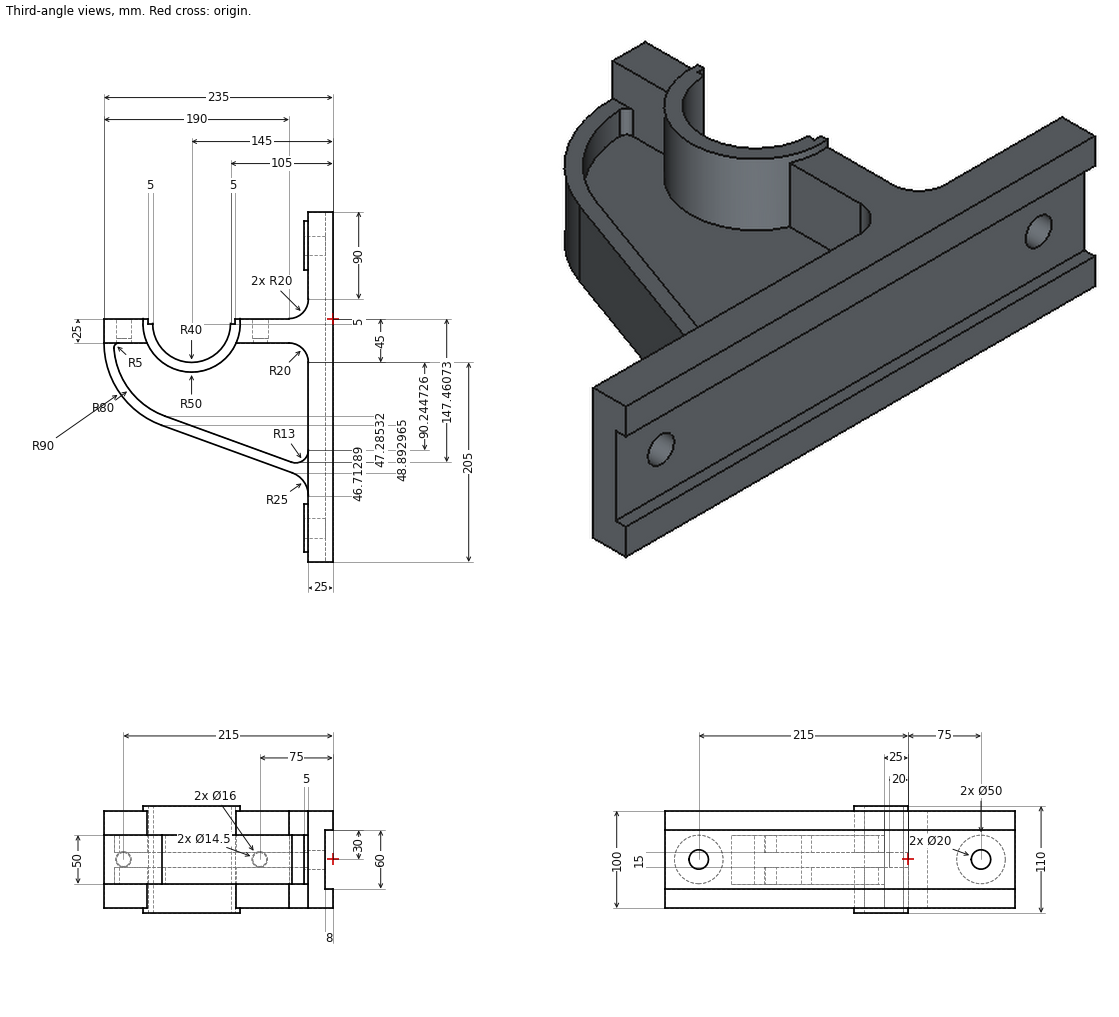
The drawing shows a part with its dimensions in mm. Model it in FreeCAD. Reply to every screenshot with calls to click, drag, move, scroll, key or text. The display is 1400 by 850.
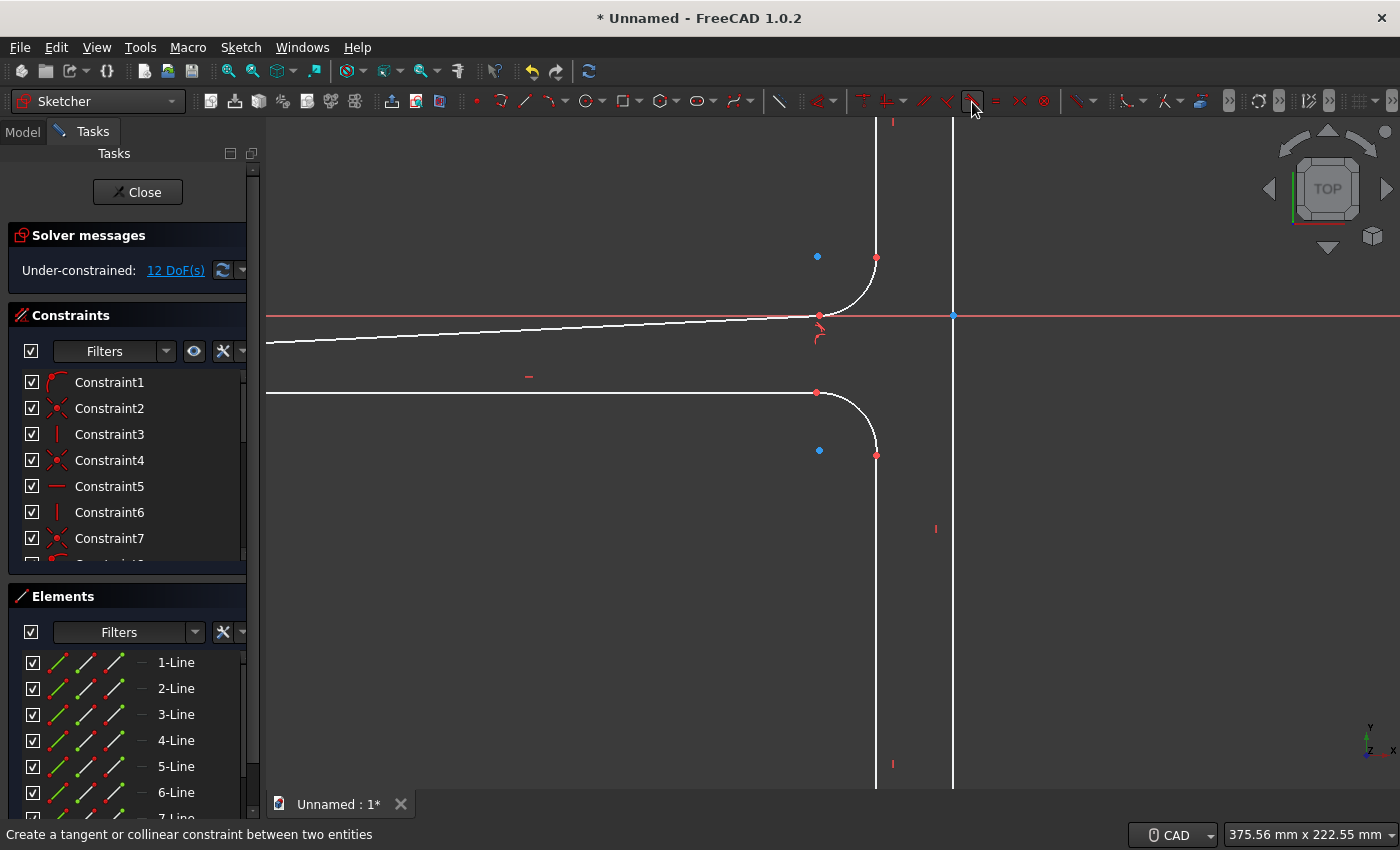
click(415, 393)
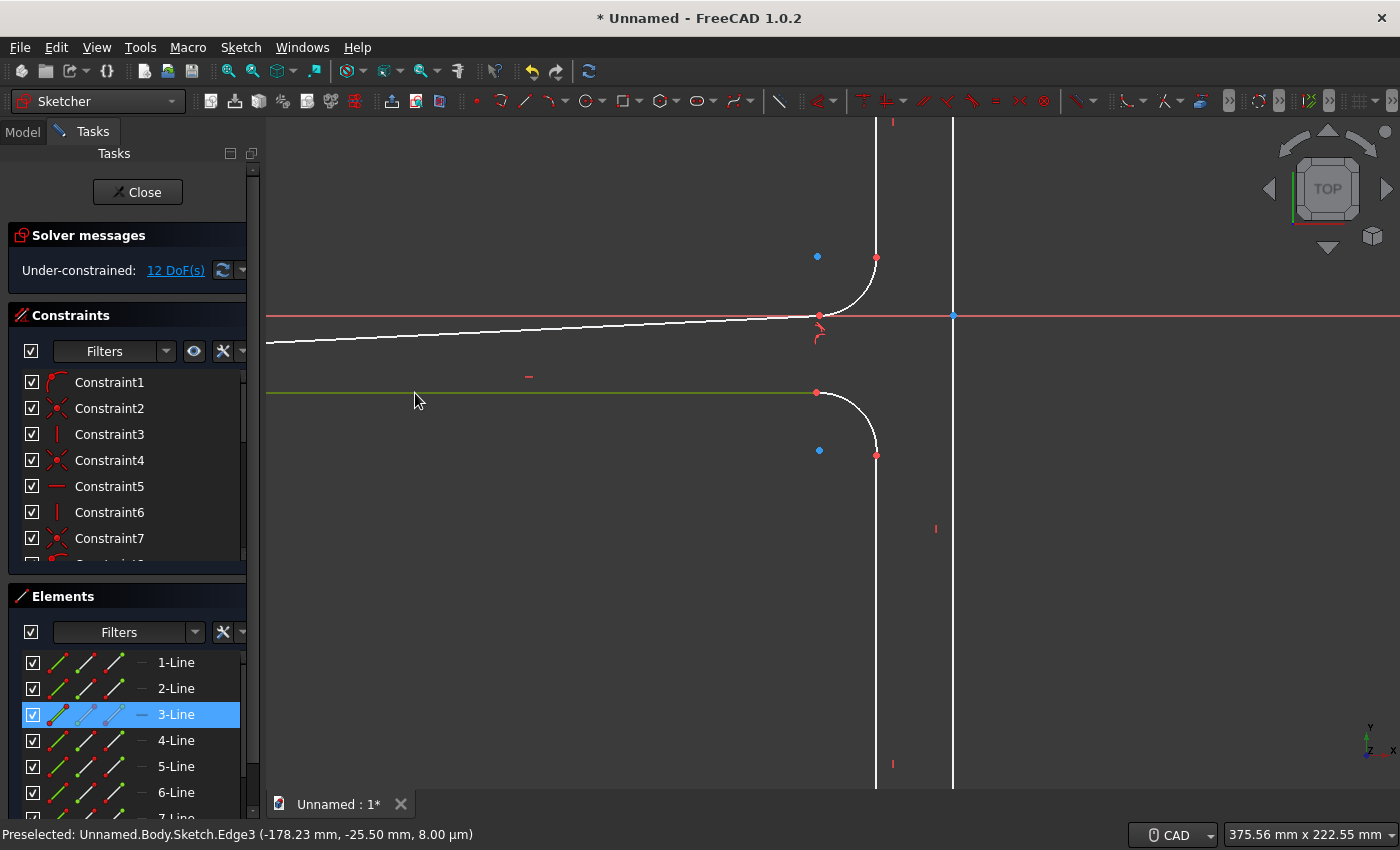
click(872, 427)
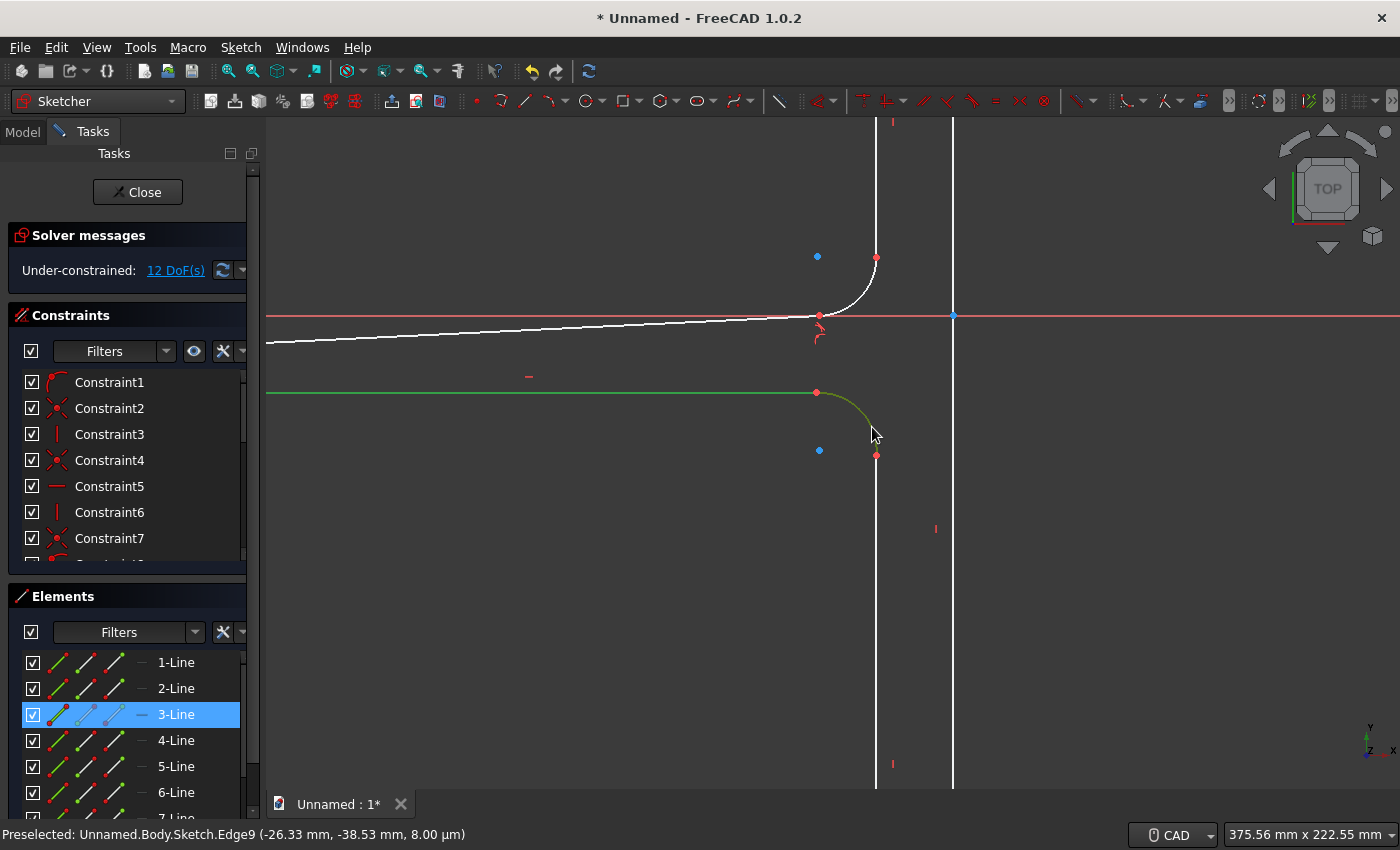
click(972, 102)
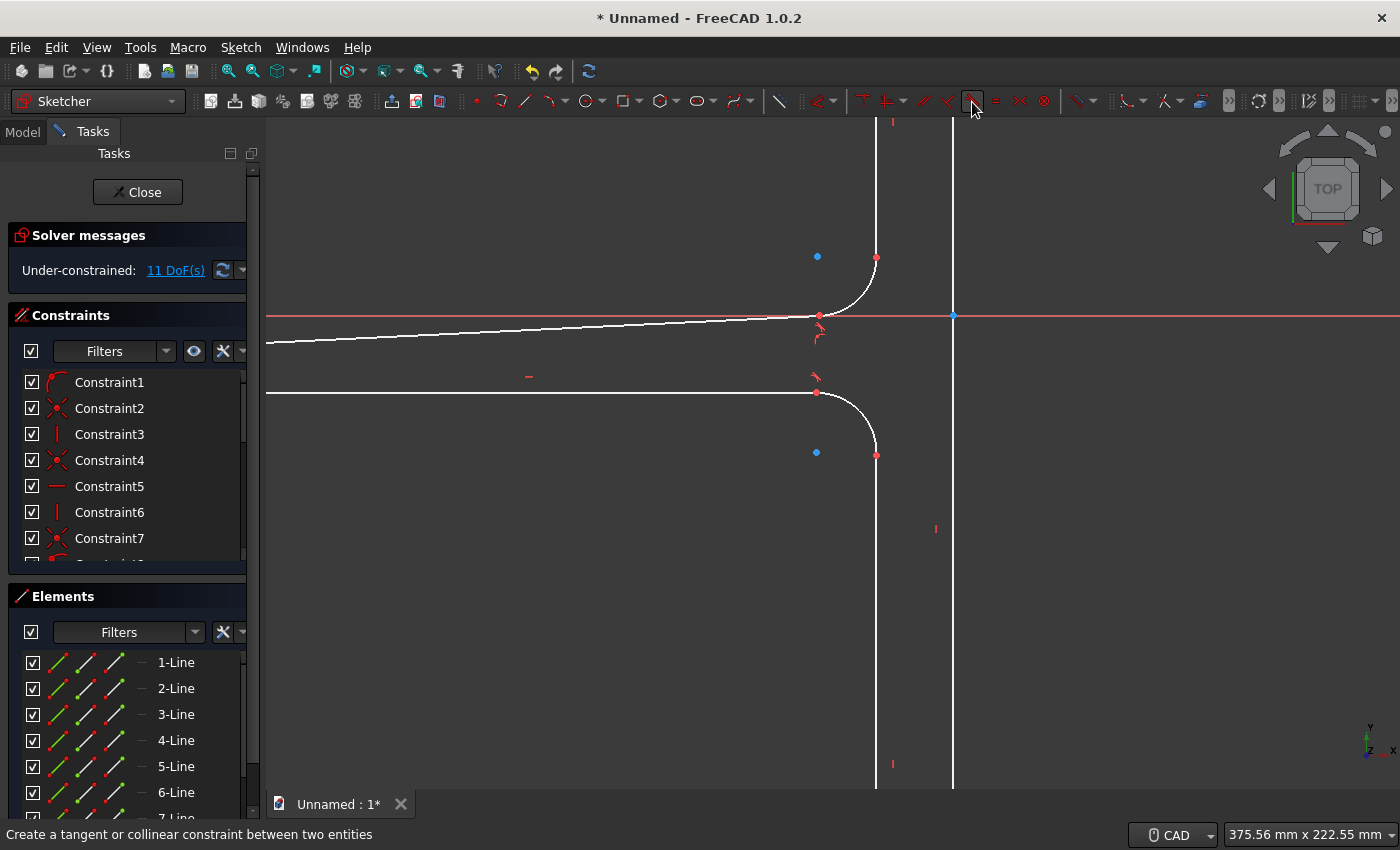
click(876, 641)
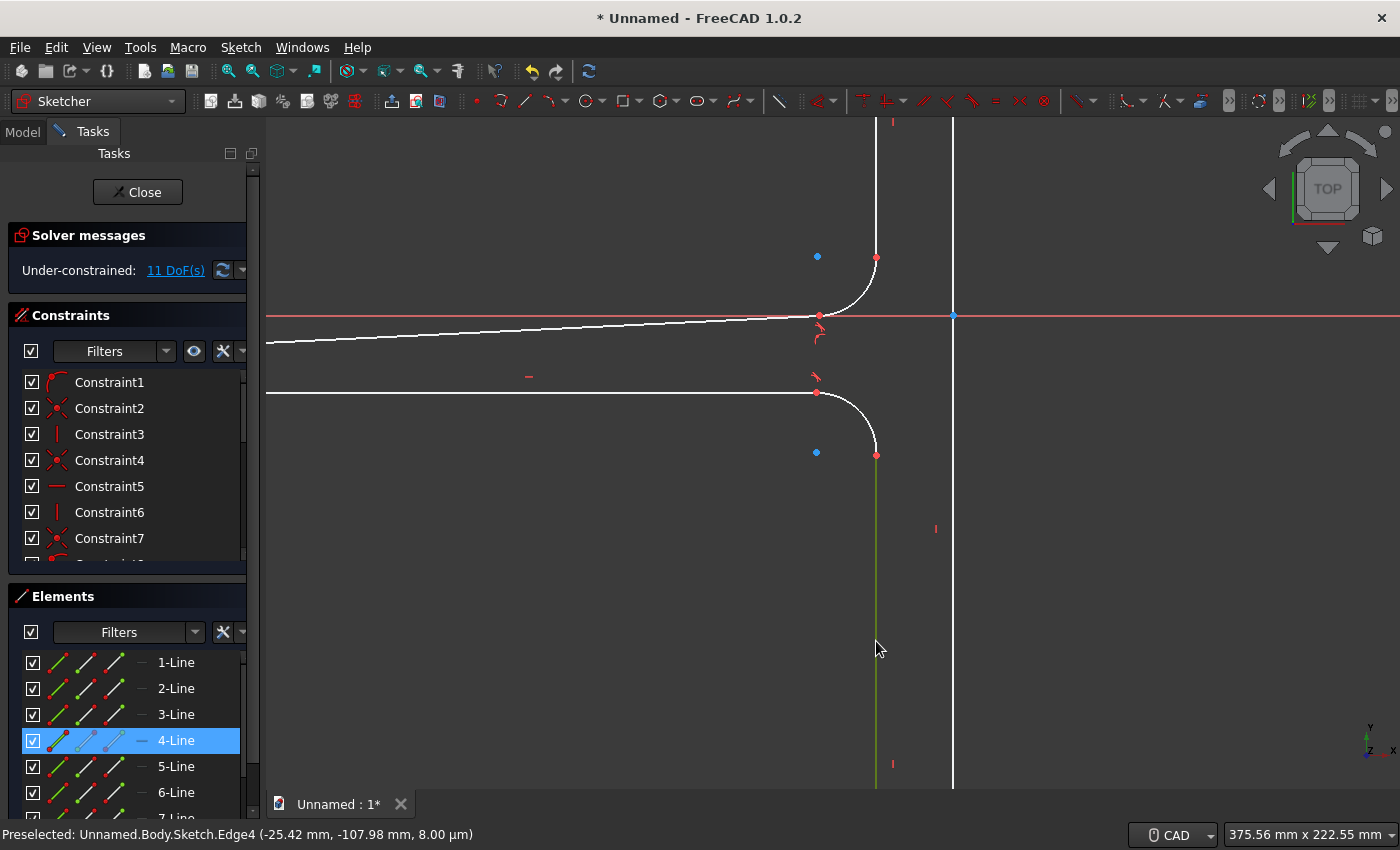
click(871, 427)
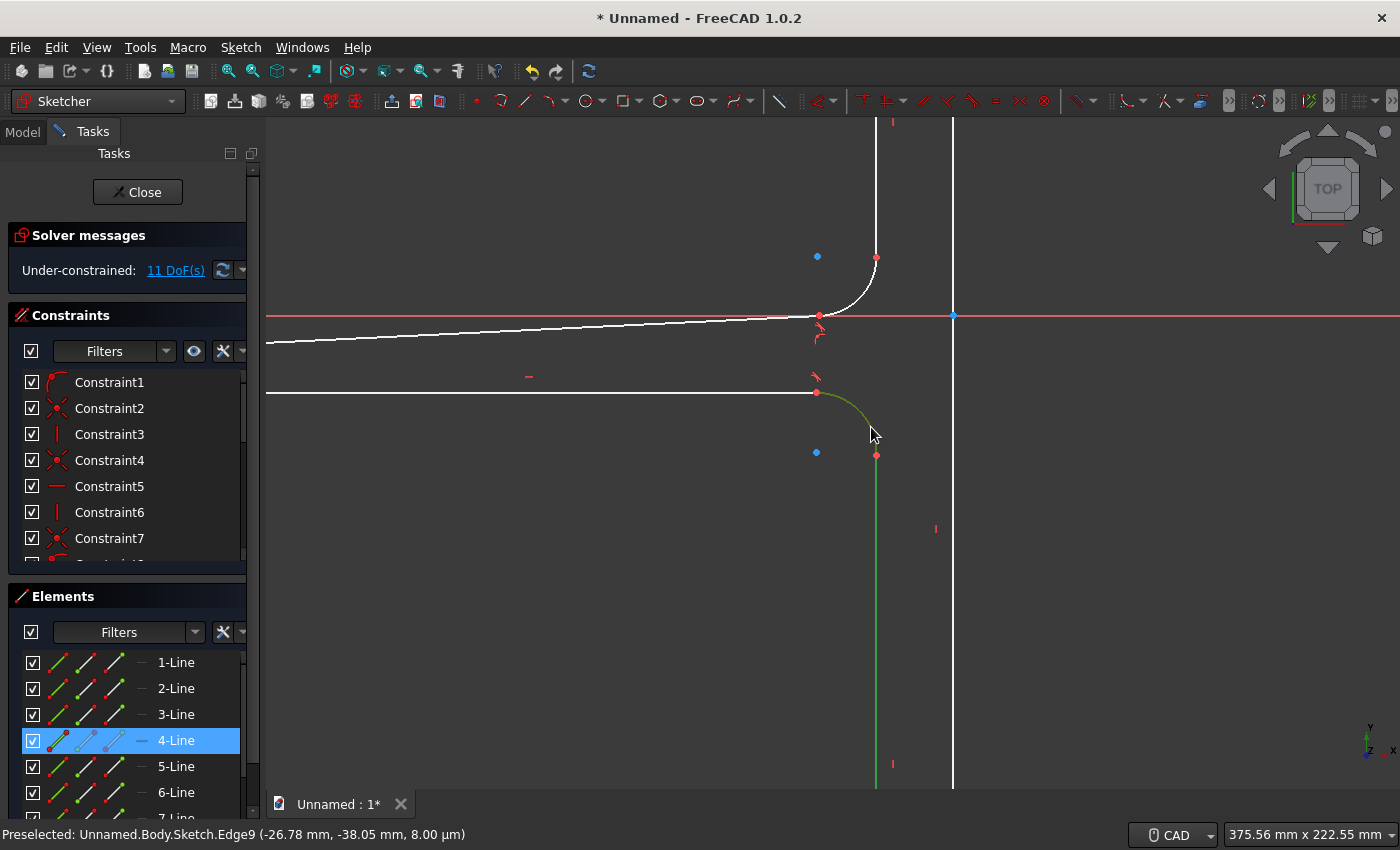
click(972, 102)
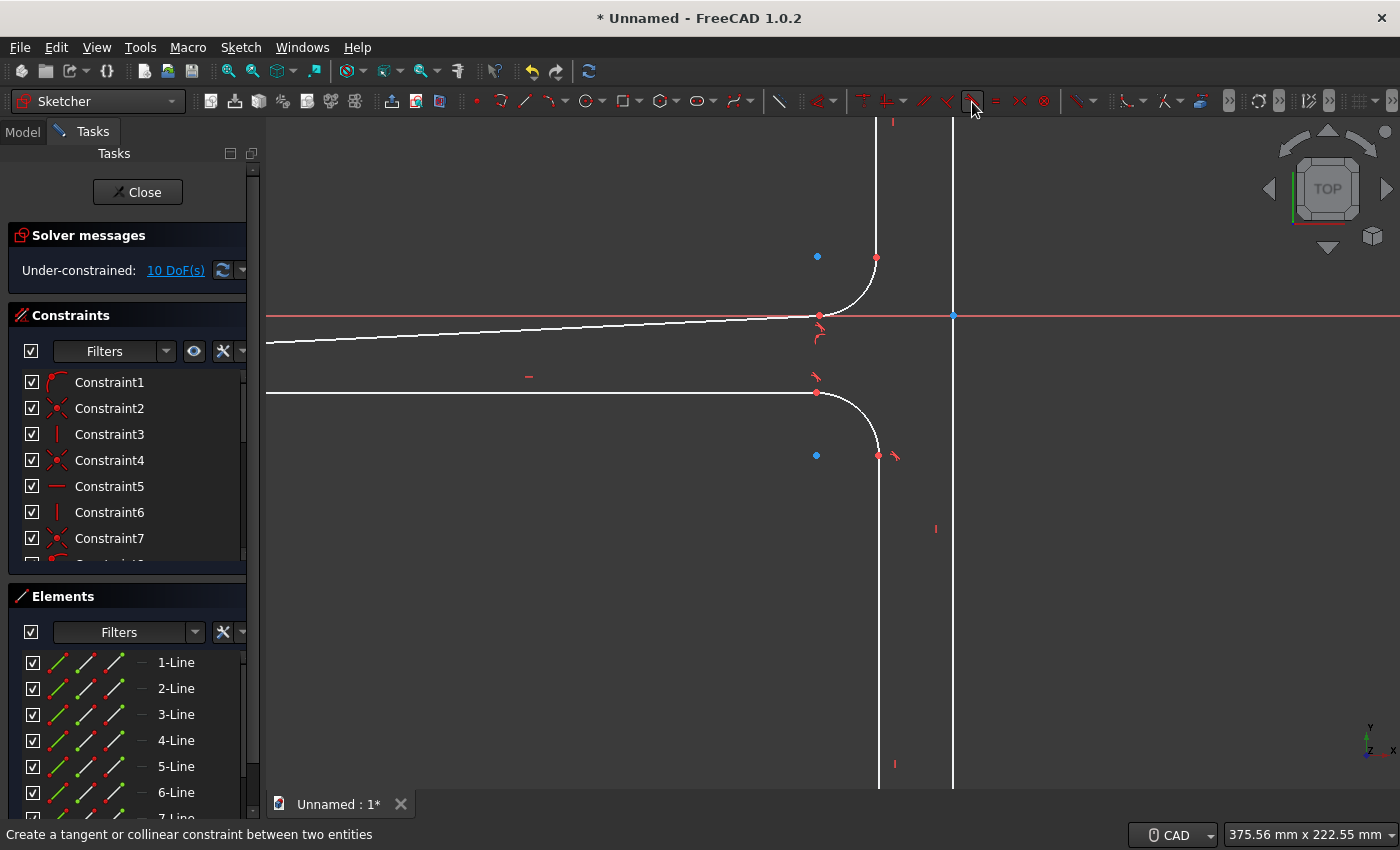
click(876, 175)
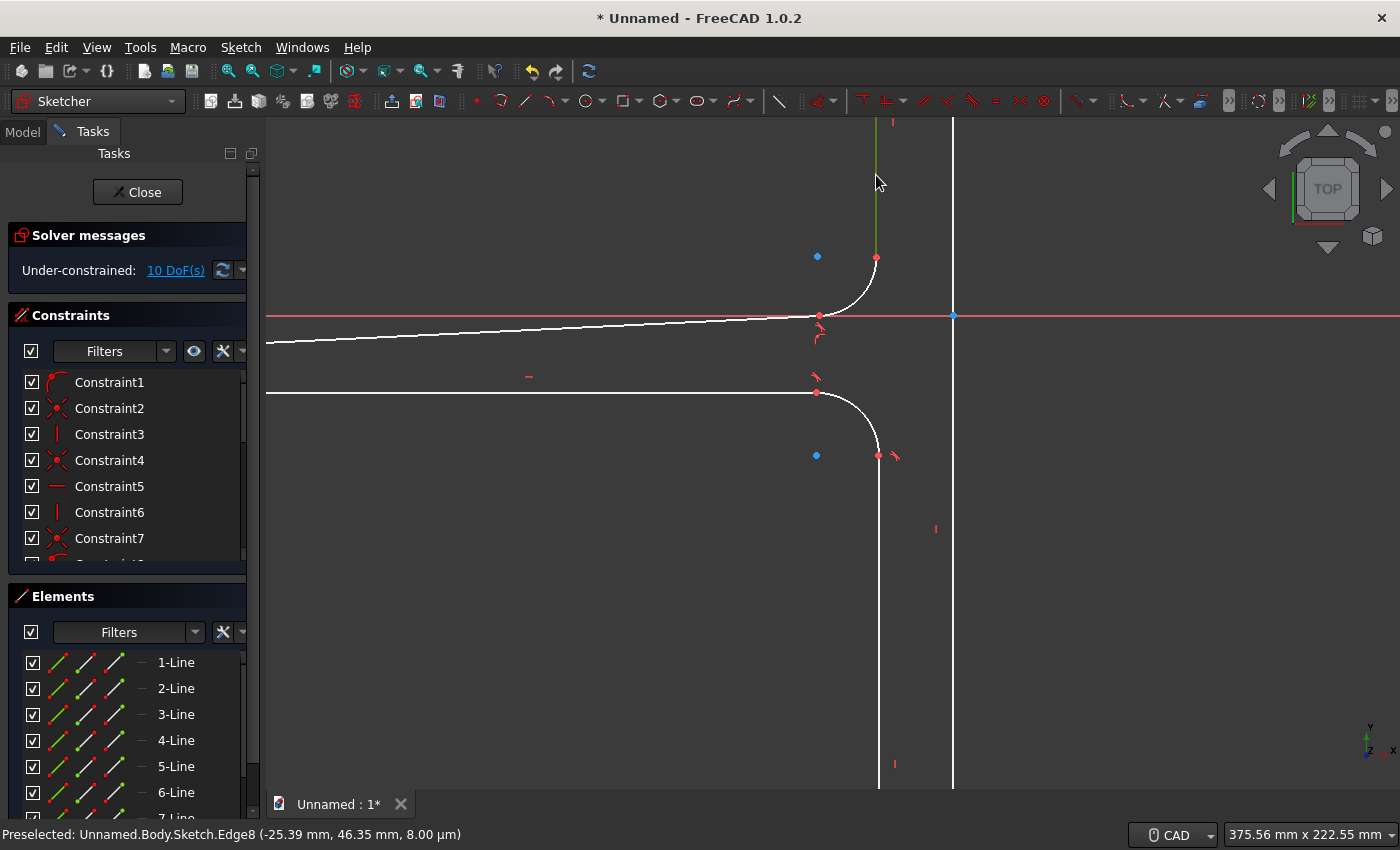
click(870, 283)